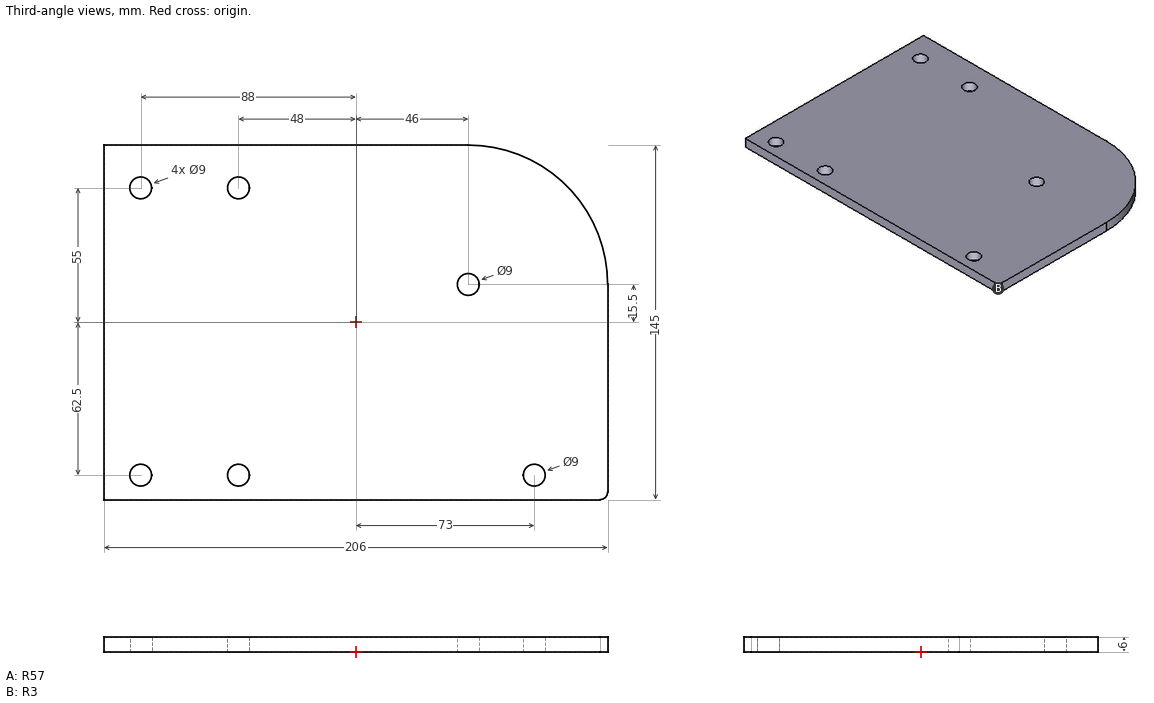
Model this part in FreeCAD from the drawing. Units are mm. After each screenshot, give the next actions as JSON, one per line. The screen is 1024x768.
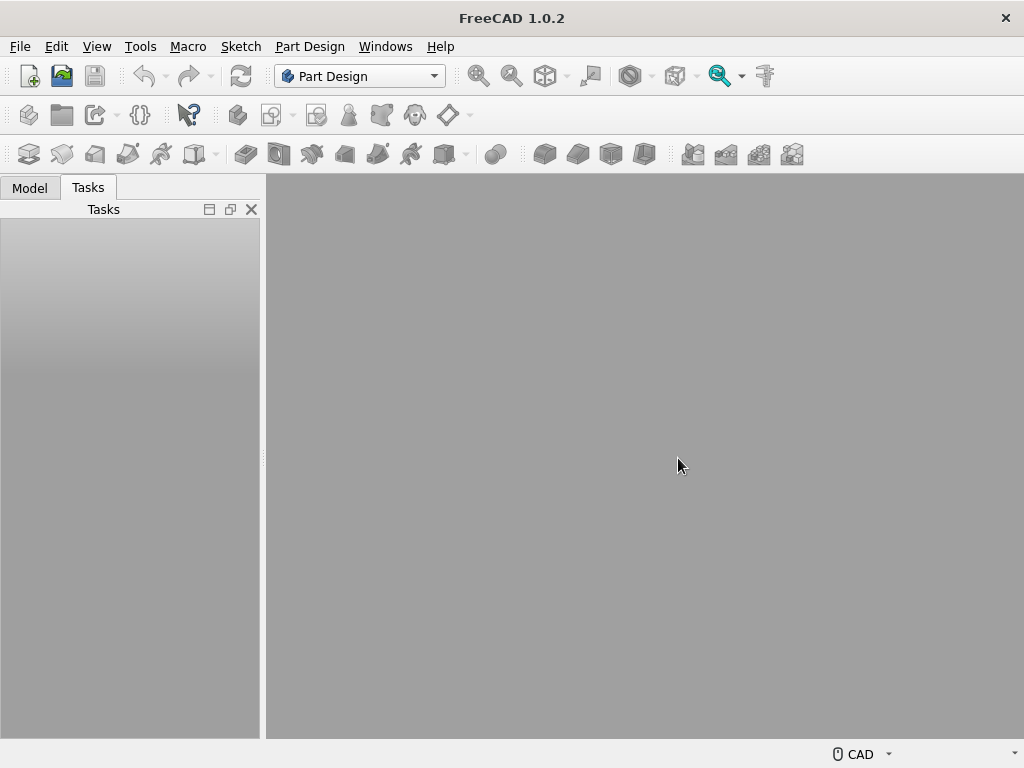
{"action": "left_click", "coordinate": [29, 76]}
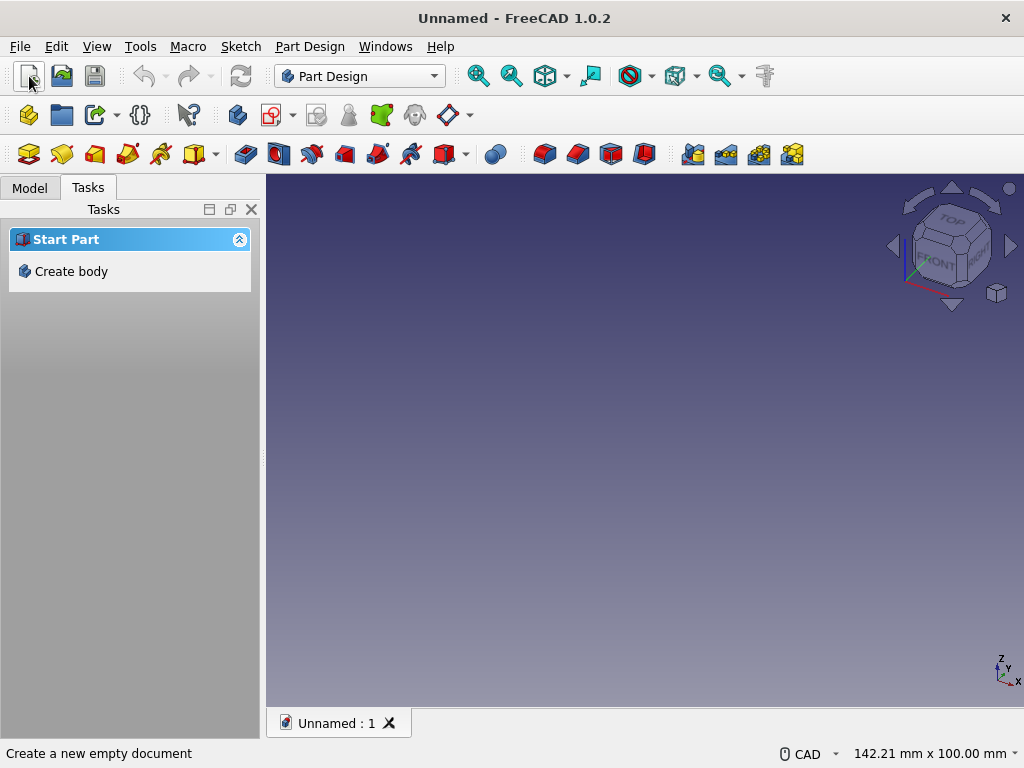
{"action": "left_click", "coordinate": [270, 116]}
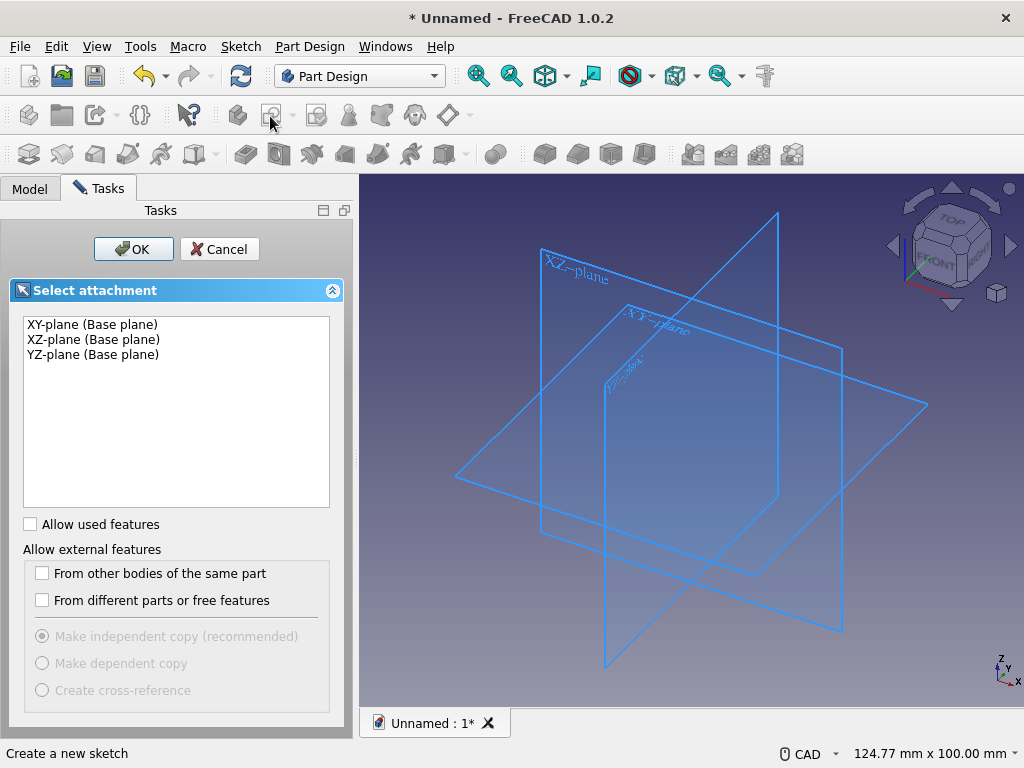
{"action": "left_click", "coordinate": [84, 324]}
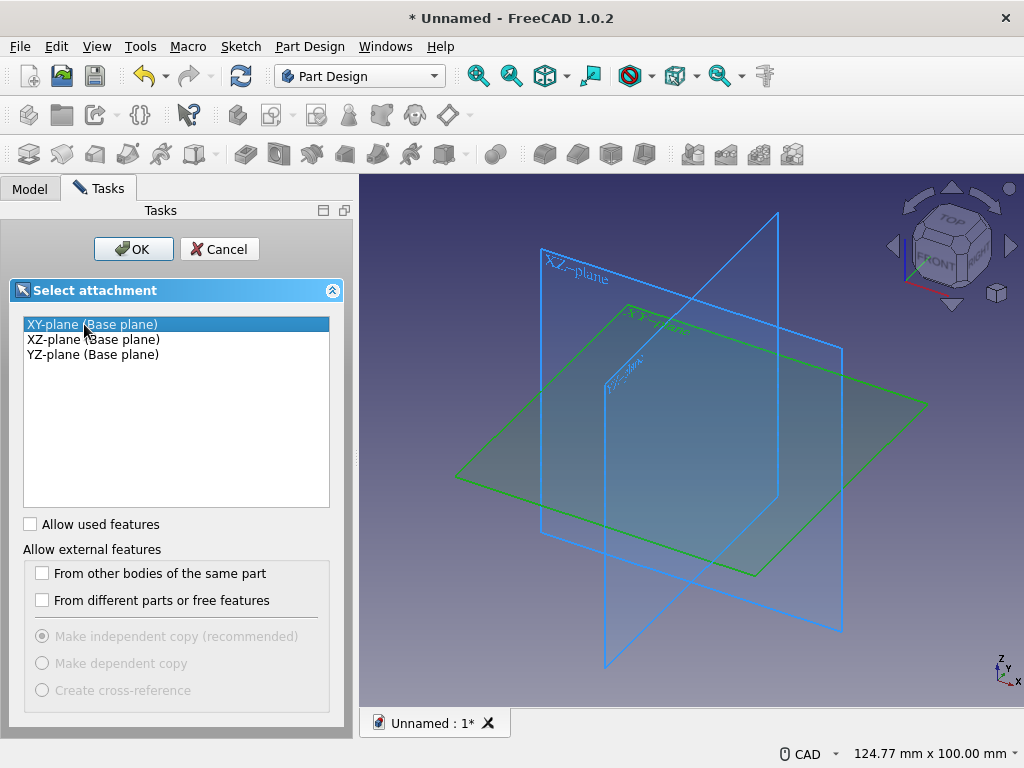
{"action": "left_click", "coordinate": [134, 249]}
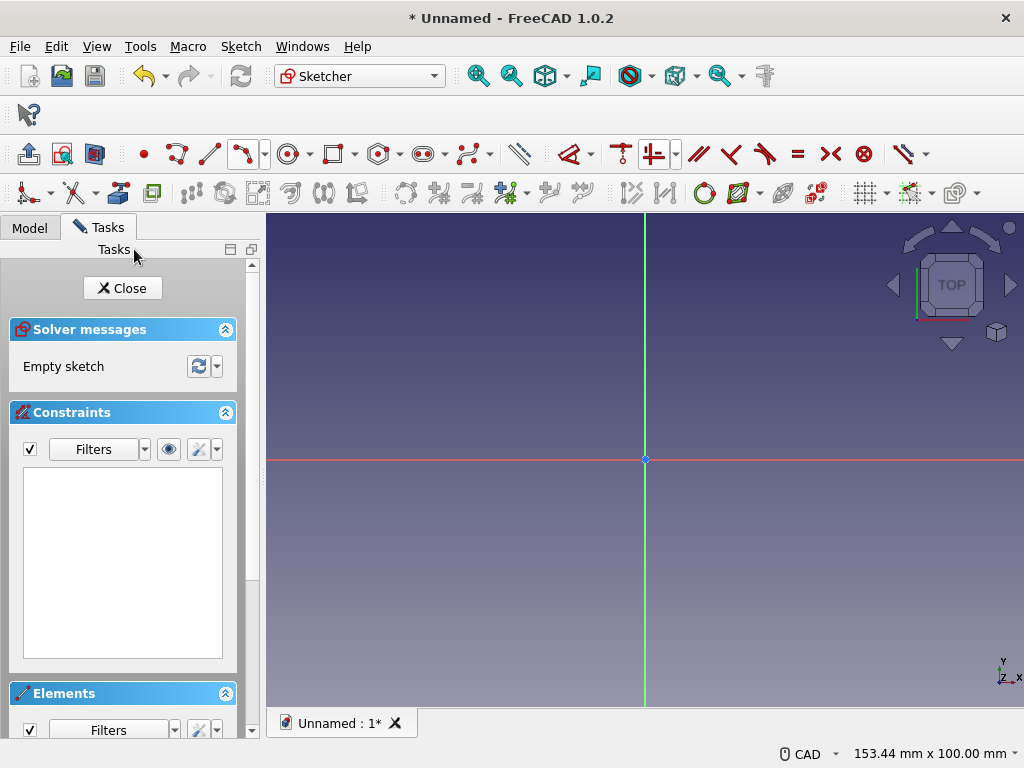
{"action": "scroll", "coordinate": [537, 460], "scroll_direction": "down", "scroll_amount": 5}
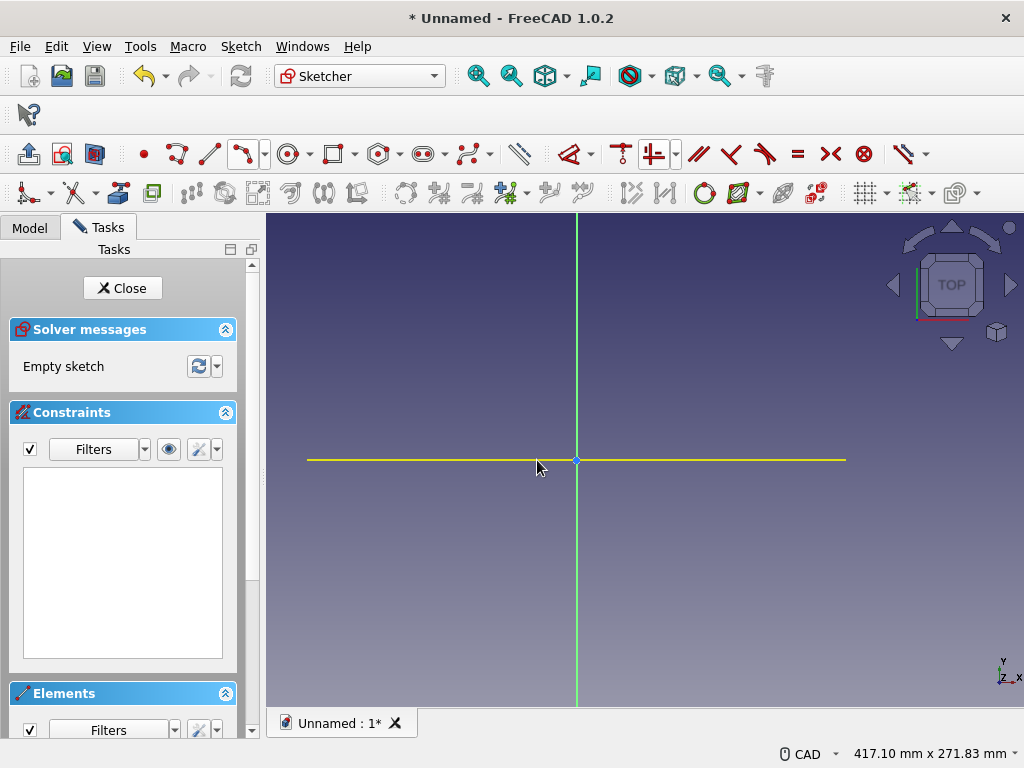
{"action": "left_click", "coordinate": [354, 154]}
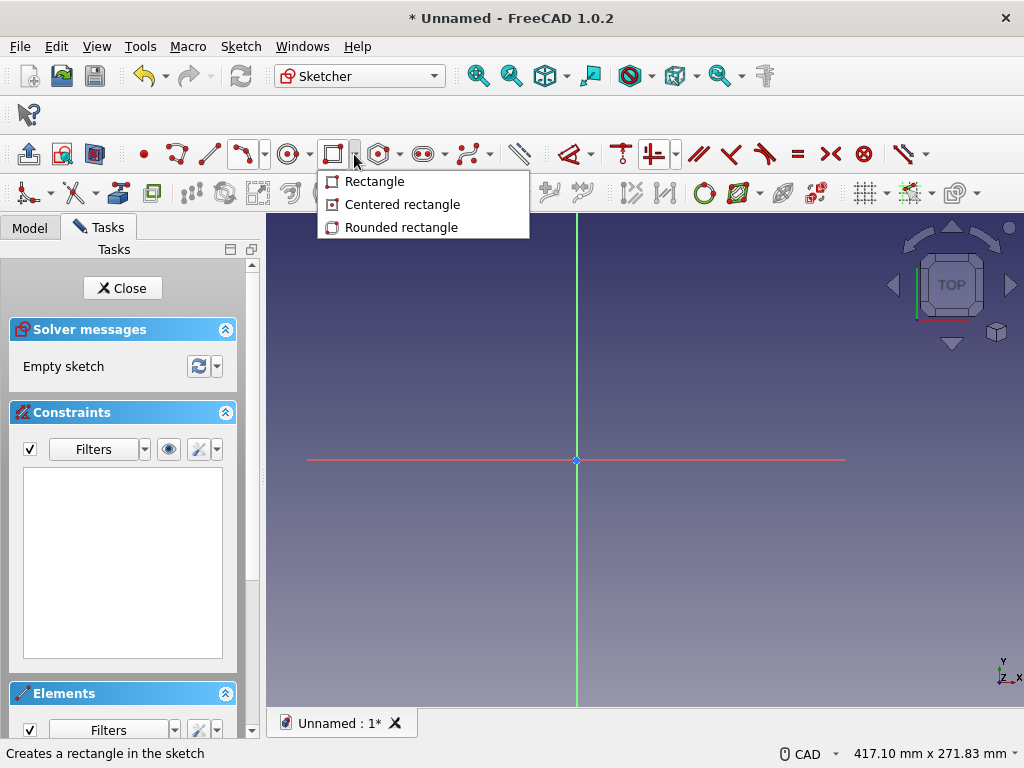
{"action": "left_click", "coordinate": [424, 204]}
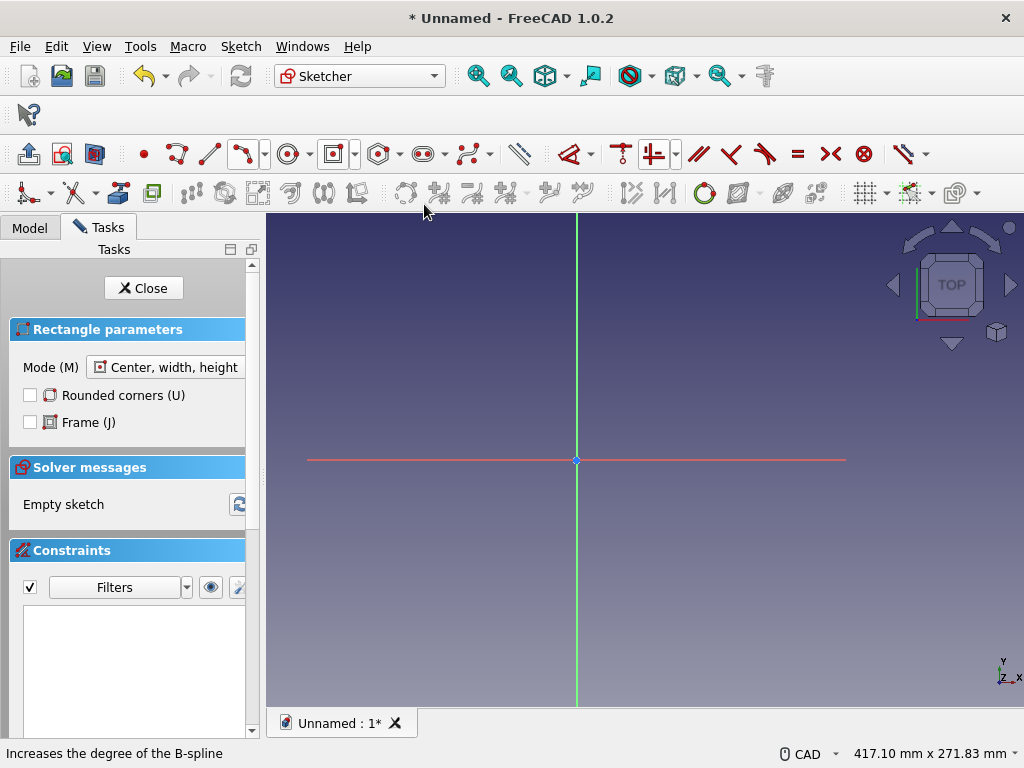
{"action": "left_click", "coordinate": [577, 460]}
{"action": "mouse_move", "coordinate": [764, 329]}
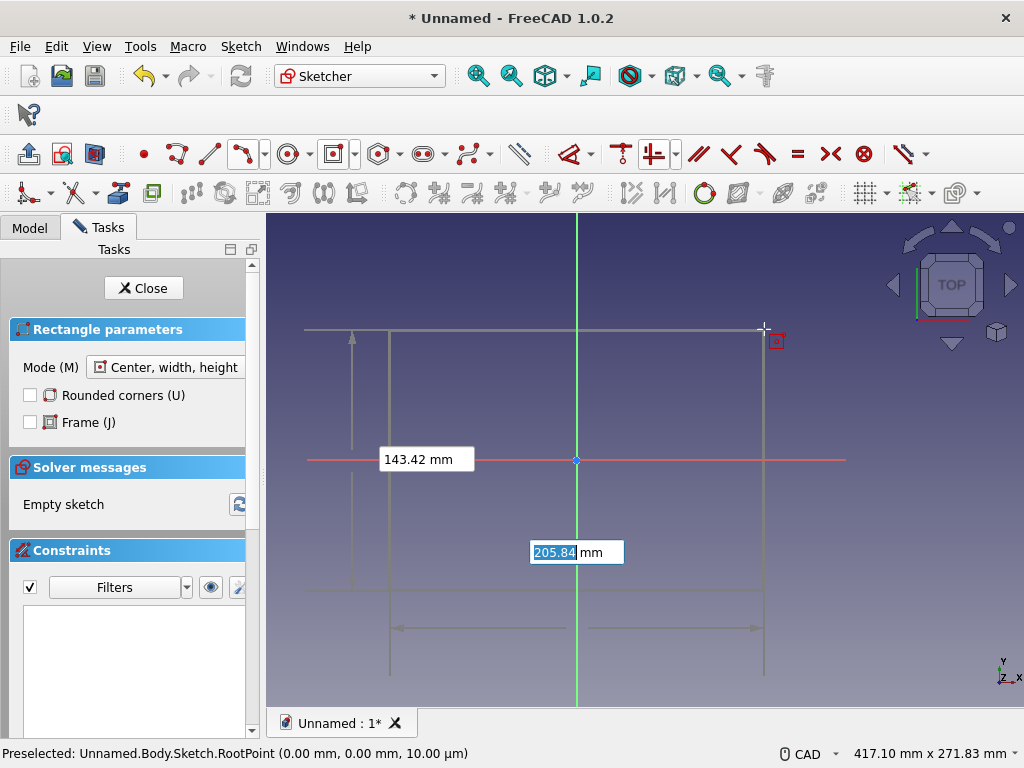
{"action": "type", "text": "206"}
{"action": "key", "text": "Tab"}
{"action": "type", "text": "145"}
{"action": "key", "text": "Return"}
{"action": "key", "text": "Escape"}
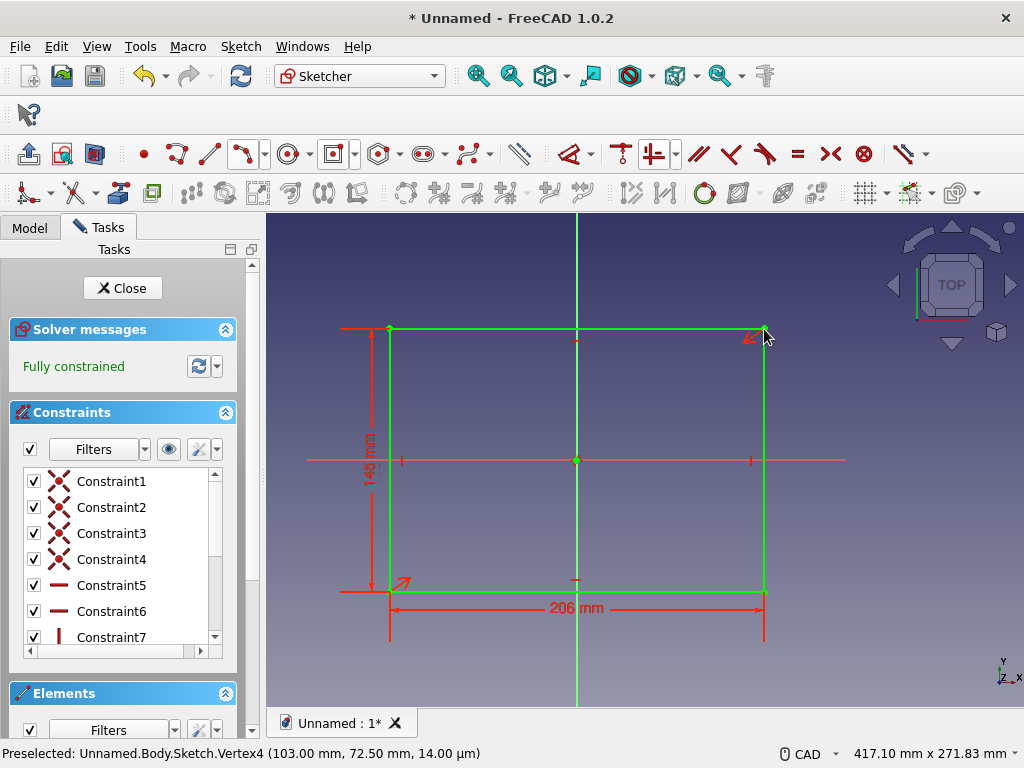
{"action": "left_click", "coordinate": [123, 288]}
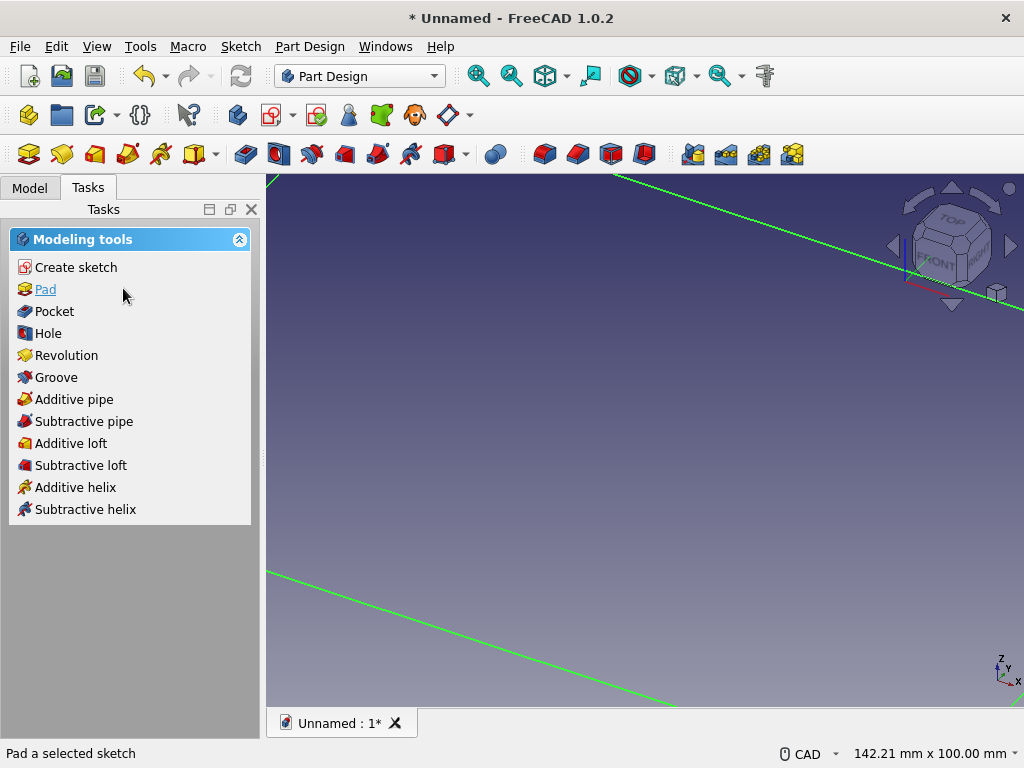
{"action": "left_click", "coordinate": [29, 154]}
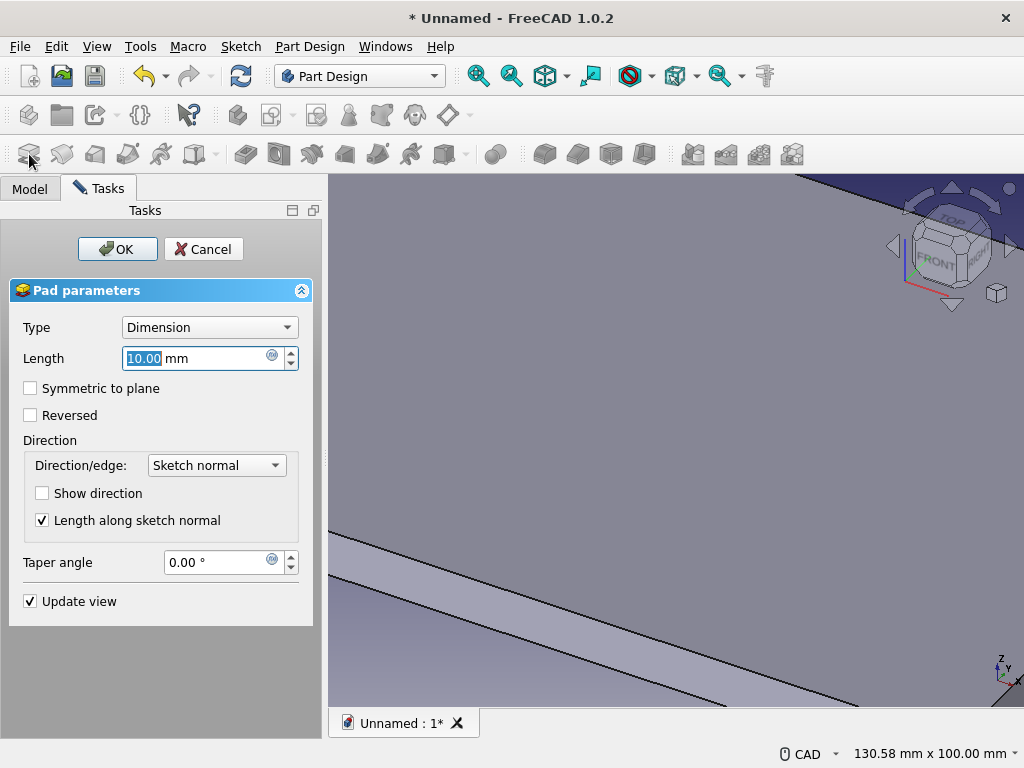
{"action": "type", "text": "6"}
{"action": "key", "text": "Tab"}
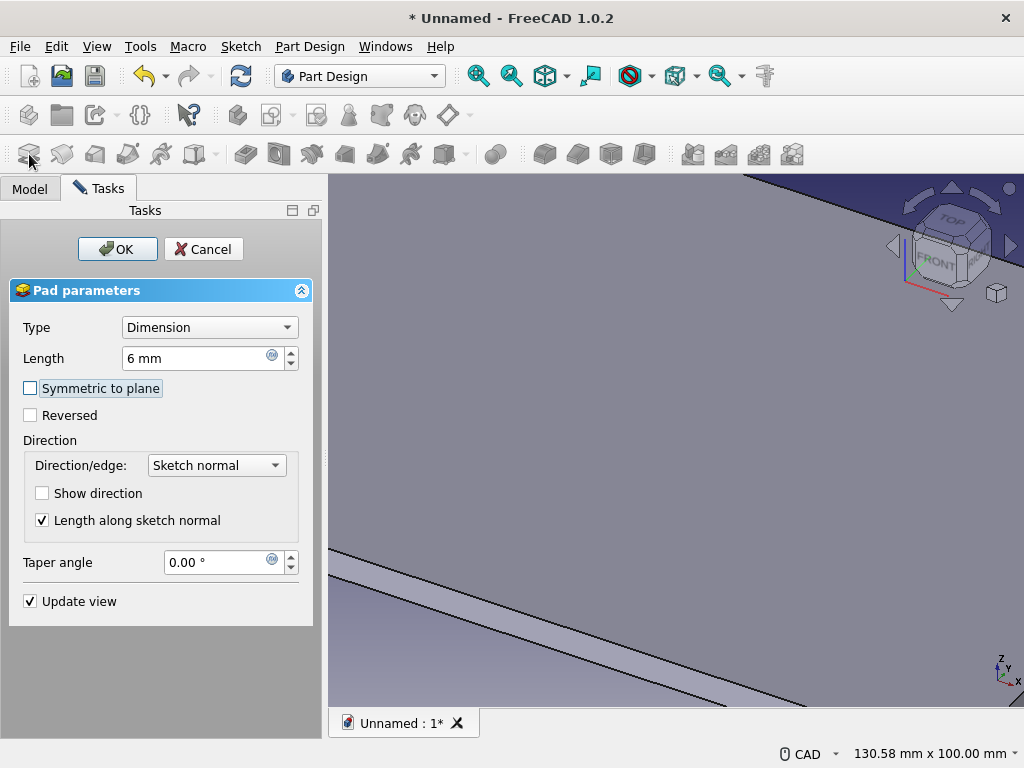
{"action": "left_click", "coordinate": [118, 249]}